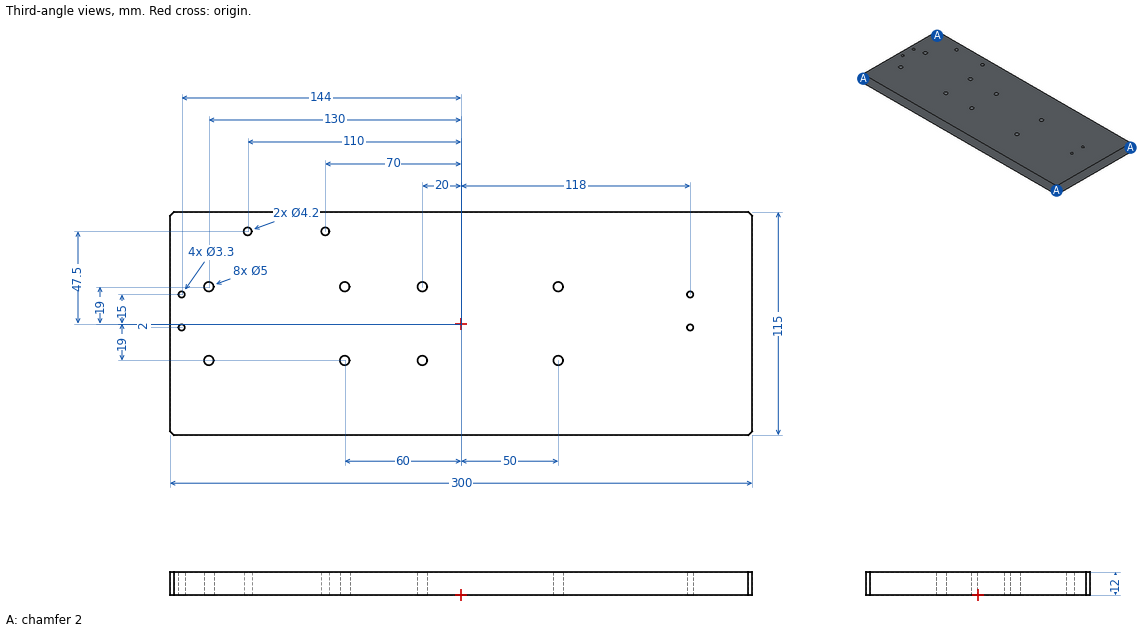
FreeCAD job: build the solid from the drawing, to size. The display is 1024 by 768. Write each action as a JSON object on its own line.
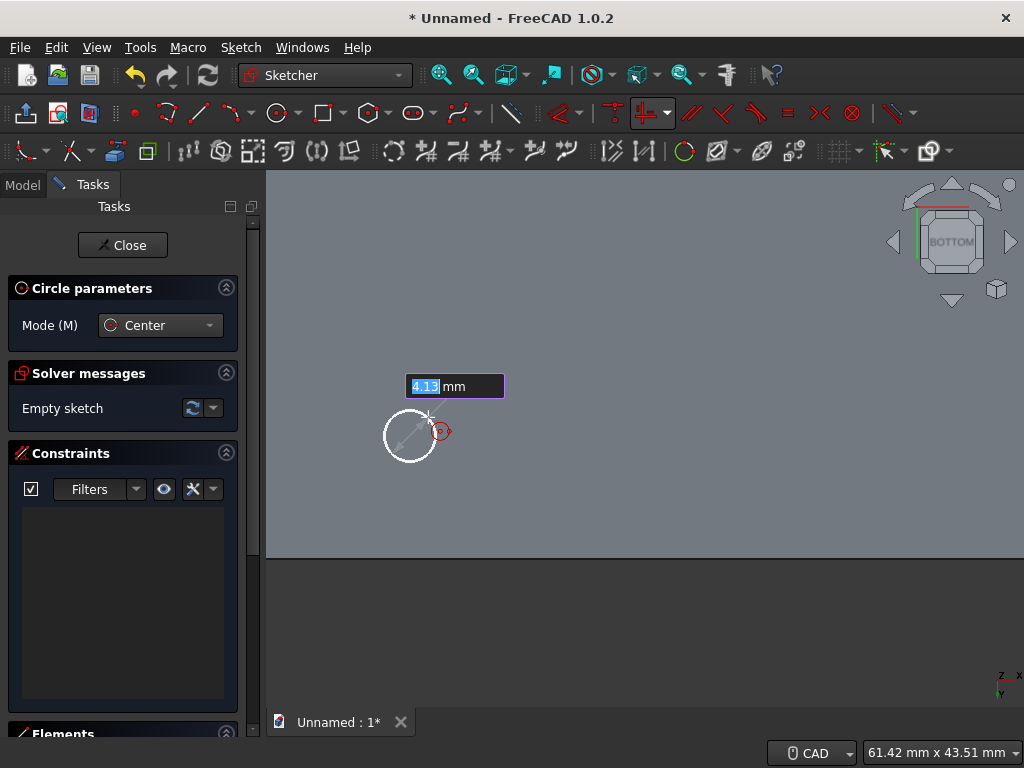
{"action": "type", "text": "4.2"}
{"action": "key", "text": "Return"}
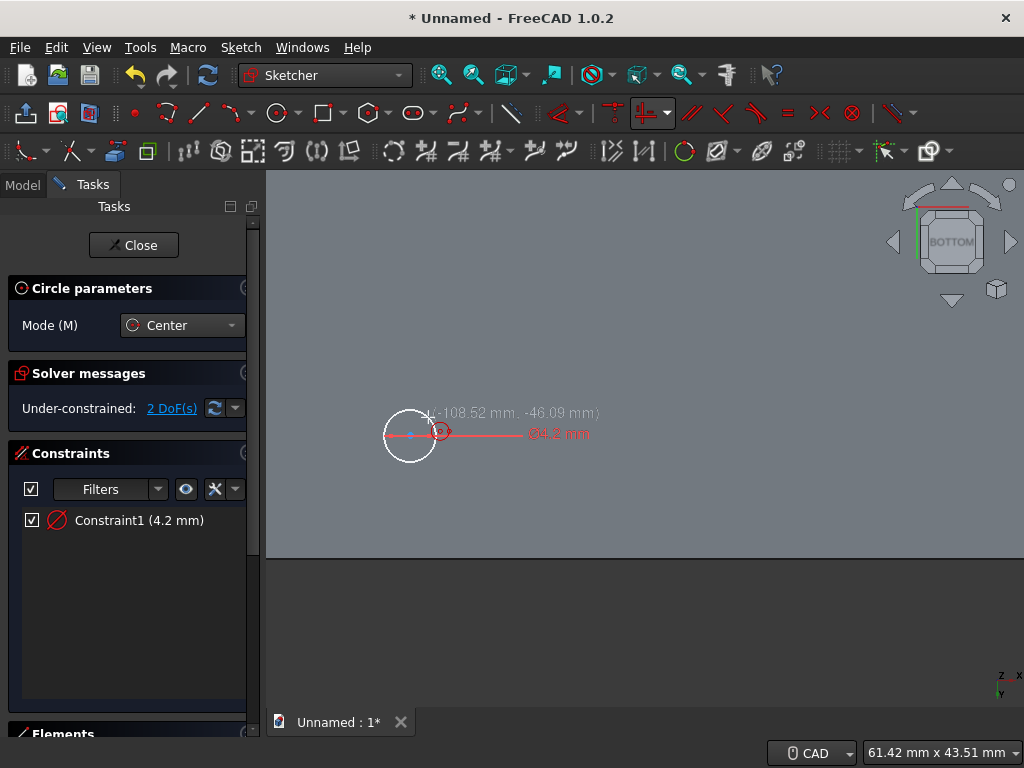
{"action": "scroll", "coordinate": [414, 445], "scroll_direction": "down", "scroll_amount": 2}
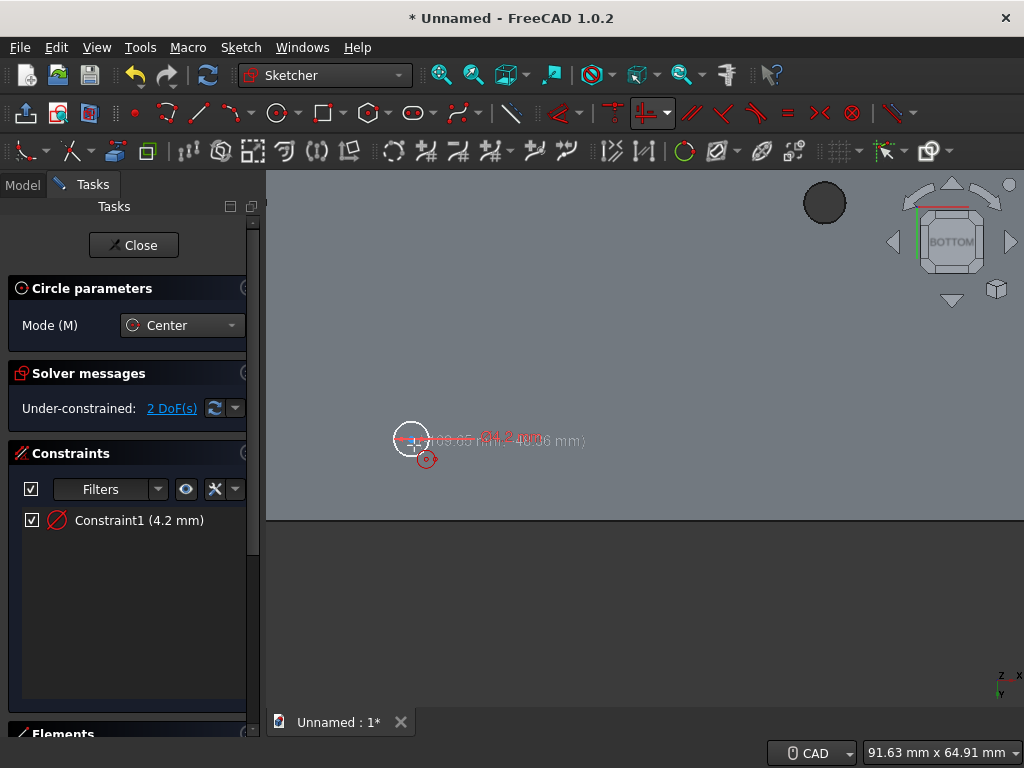
{"action": "scroll", "coordinate": [742, 439], "scroll_direction": "up", "scroll_amount": 2}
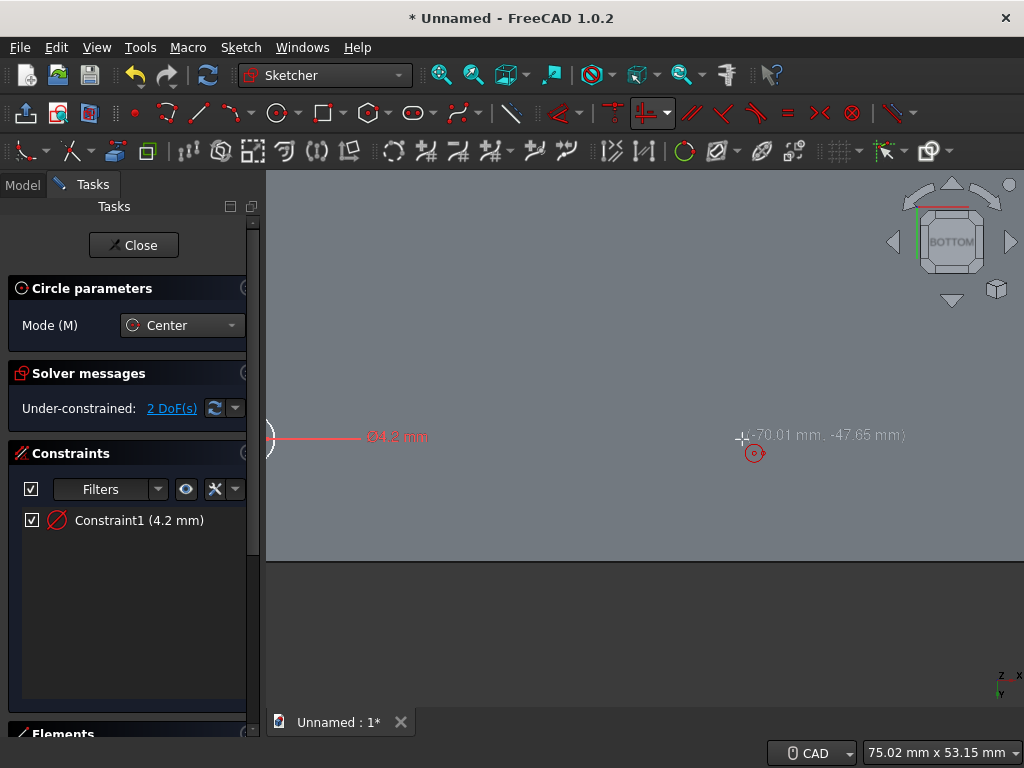
{"action": "left_click", "coordinate": [742, 438]}
{"action": "mouse_move", "coordinate": [760, 420]}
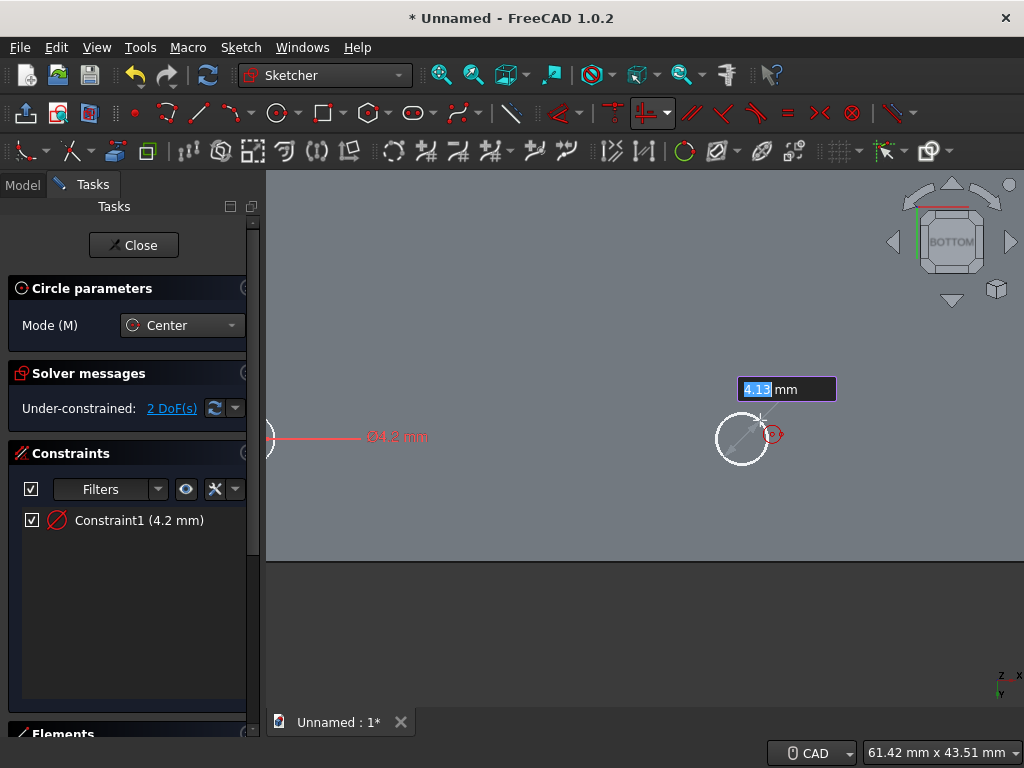
{"action": "type", "text": "4.2"}
{"action": "key", "text": "Return"}
{"action": "key", "text": "Escape"}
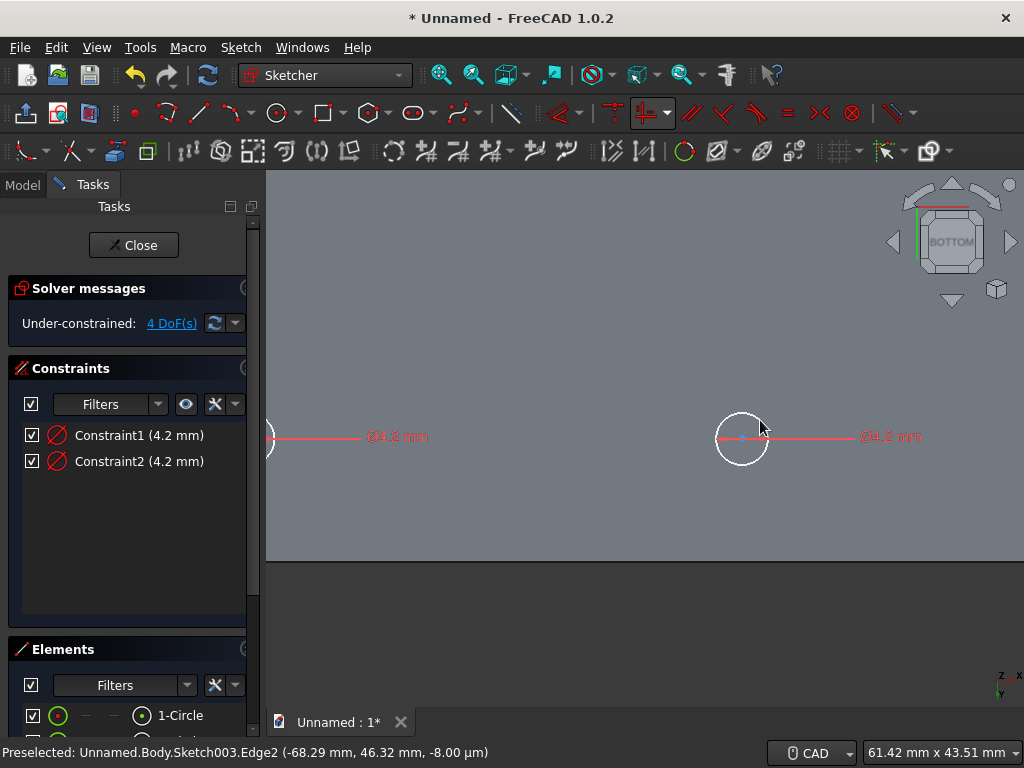
{"action": "scroll", "coordinate": [742, 439], "scroll_direction": "down", "scroll_amount": 2}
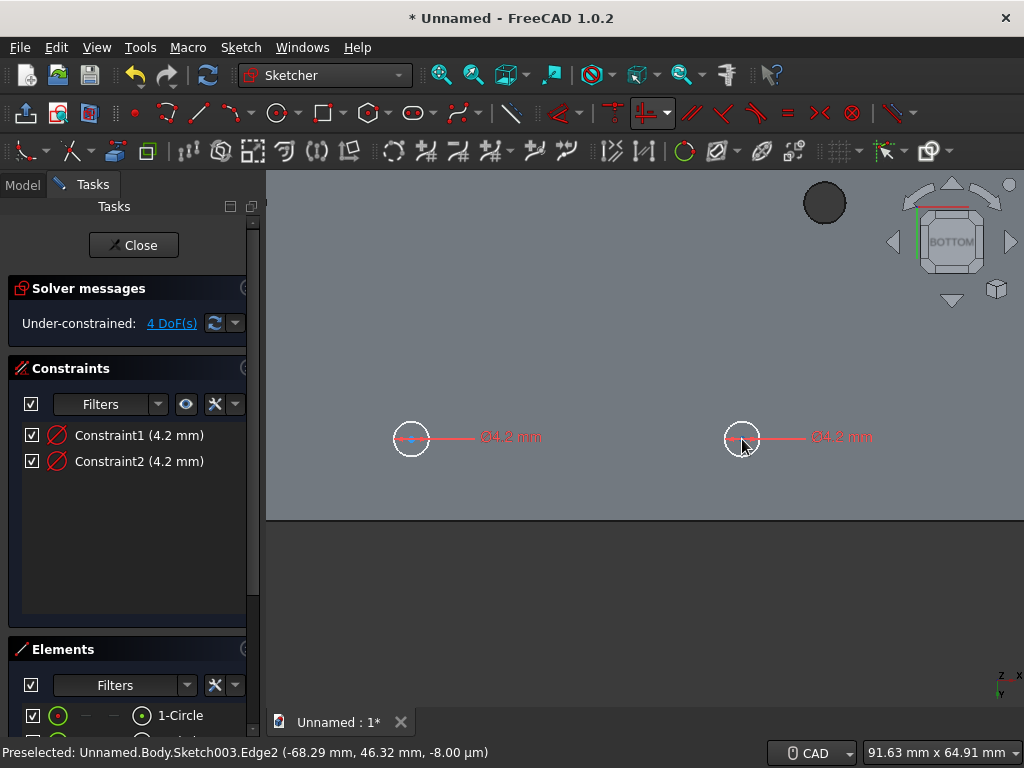
{"action": "left_click", "coordinate": [411, 439]}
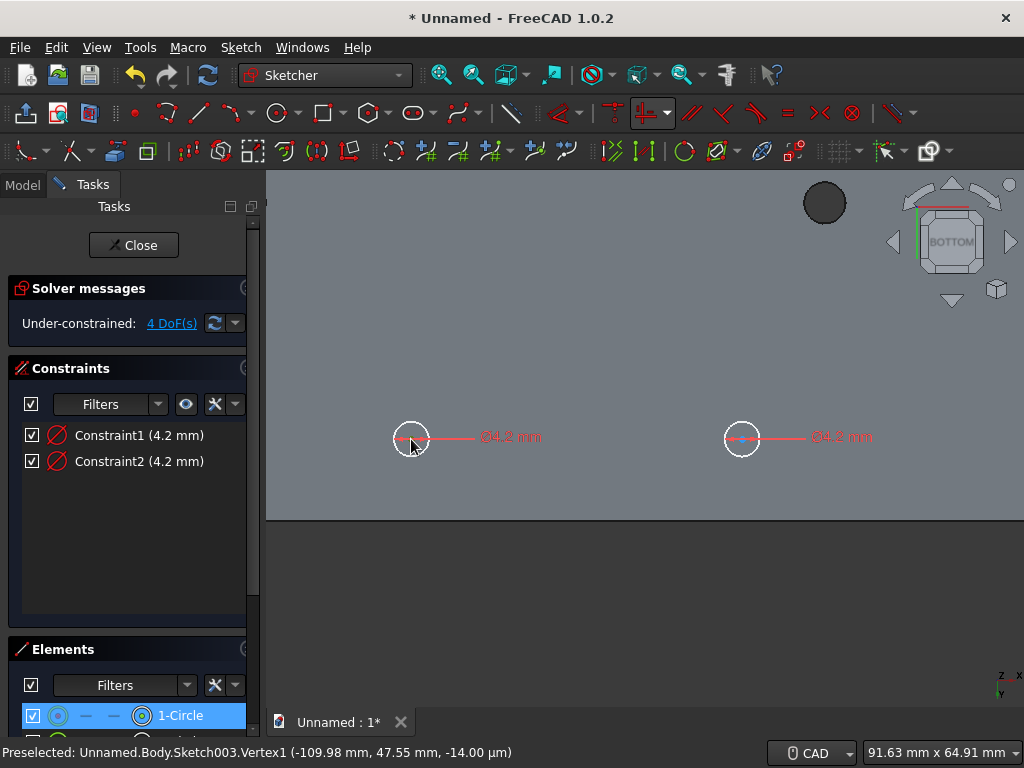
{"action": "left_click", "coordinate": [742, 439]}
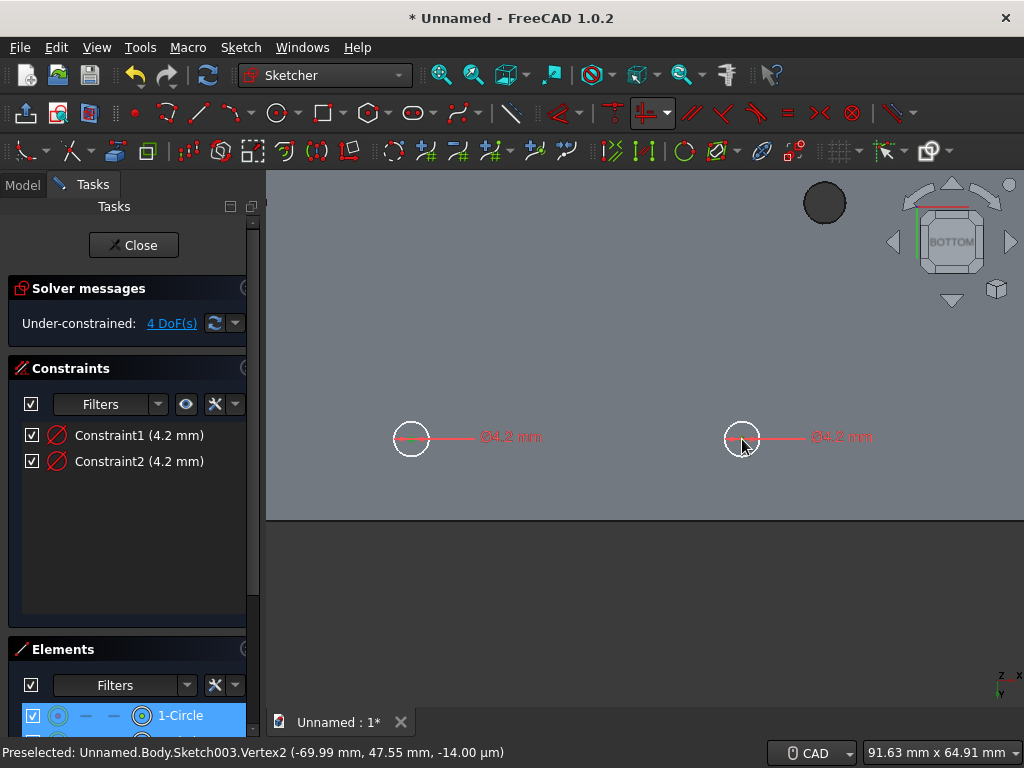
{"action": "key", "text": "h"}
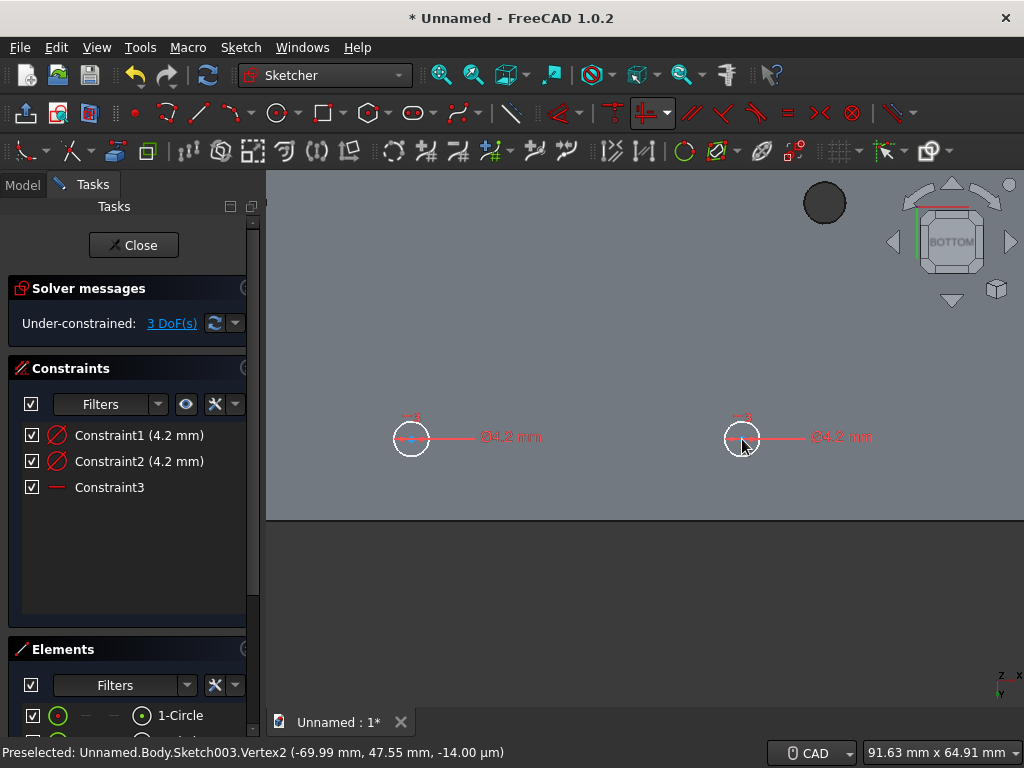
{"action": "left_click", "coordinate": [558, 114]}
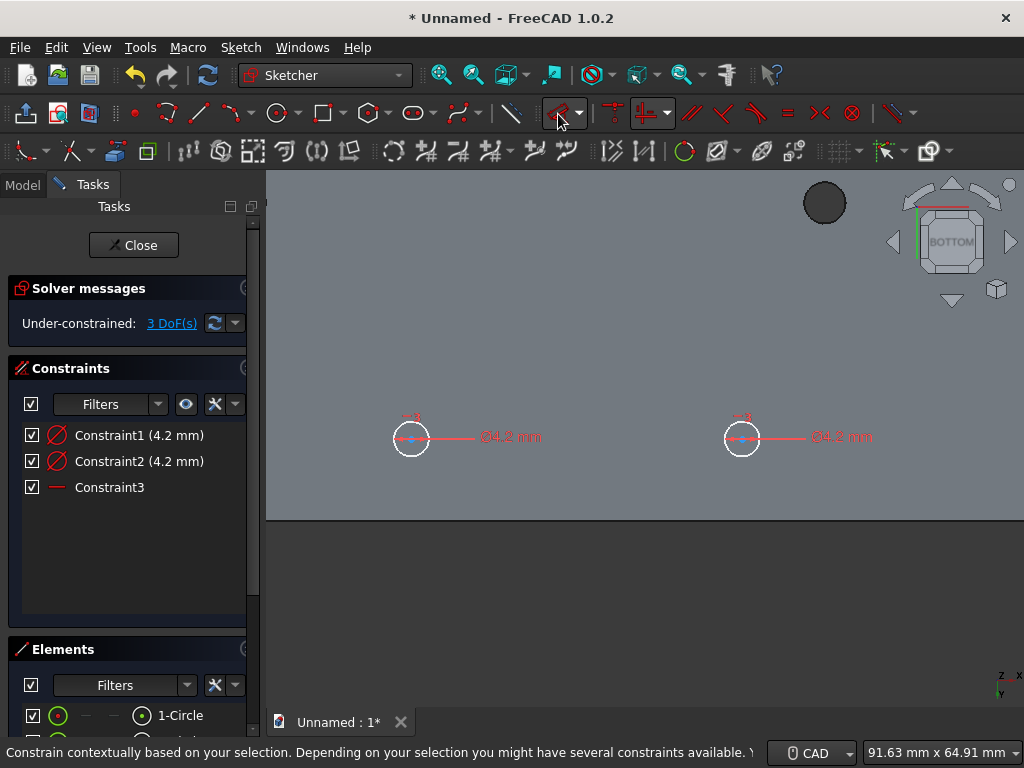
{"action": "left_click", "coordinate": [742, 439]}
{"action": "left_click", "coordinate": [801, 473]}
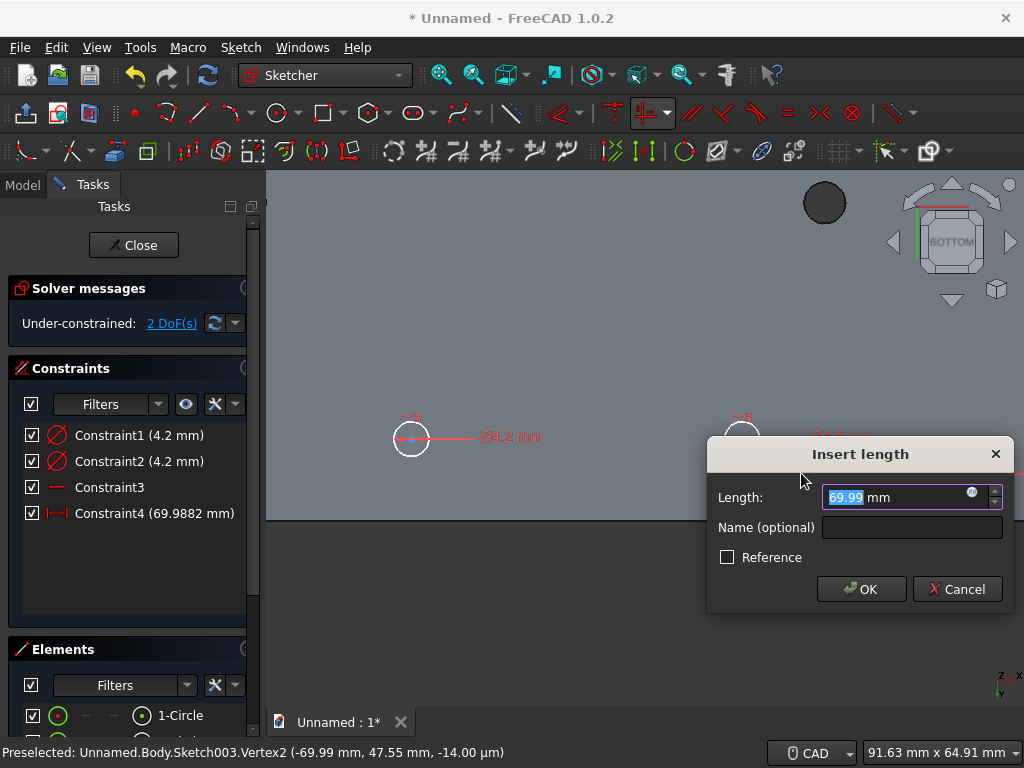
{"action": "type", "text": "70"}
{"action": "key", "text": "Return"}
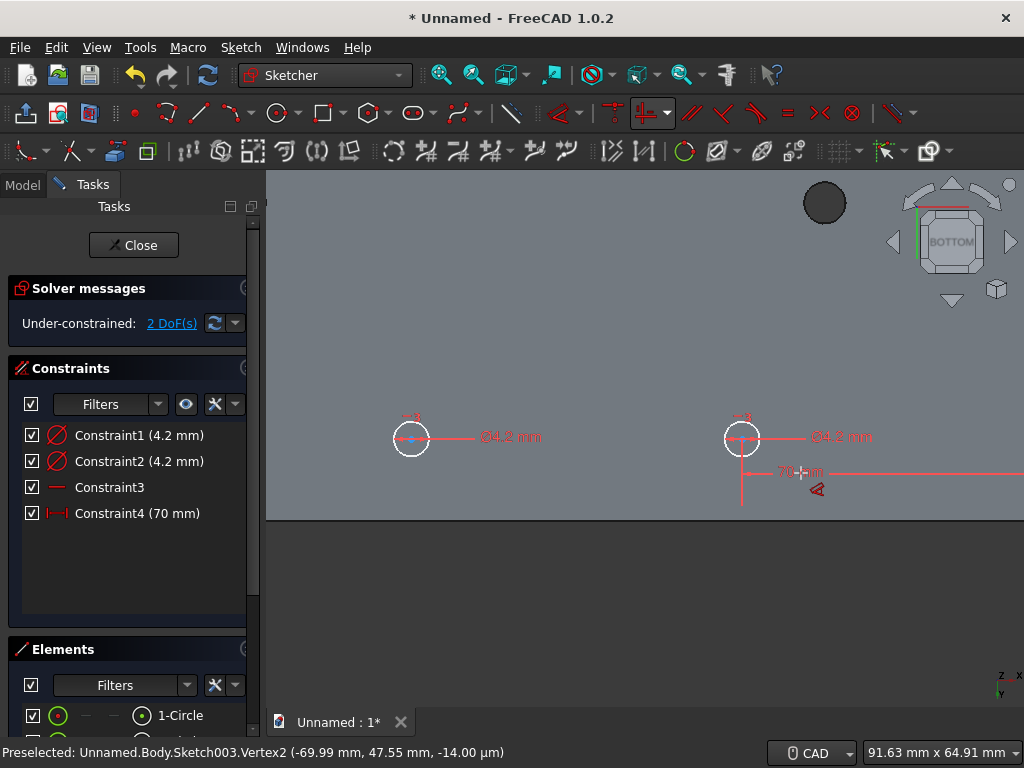
{"action": "left_click", "coordinate": [411, 439]}
{"action": "left_click", "coordinate": [635, 473]}